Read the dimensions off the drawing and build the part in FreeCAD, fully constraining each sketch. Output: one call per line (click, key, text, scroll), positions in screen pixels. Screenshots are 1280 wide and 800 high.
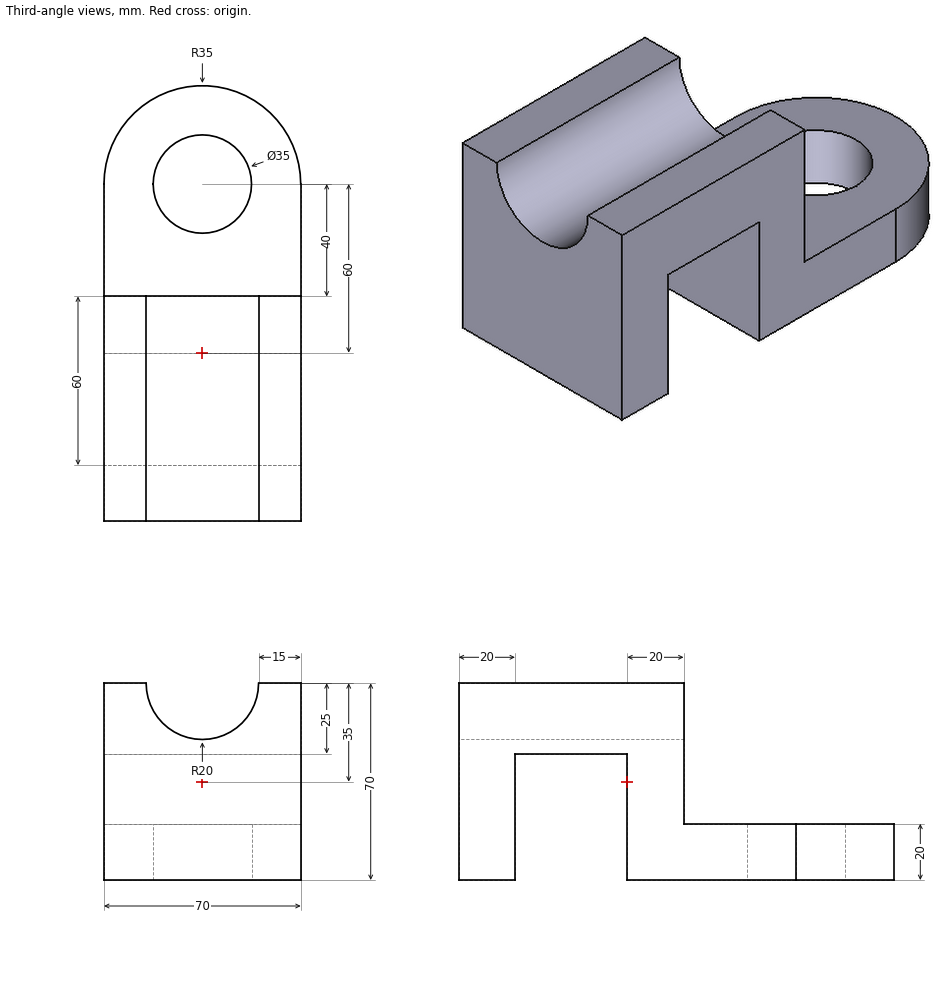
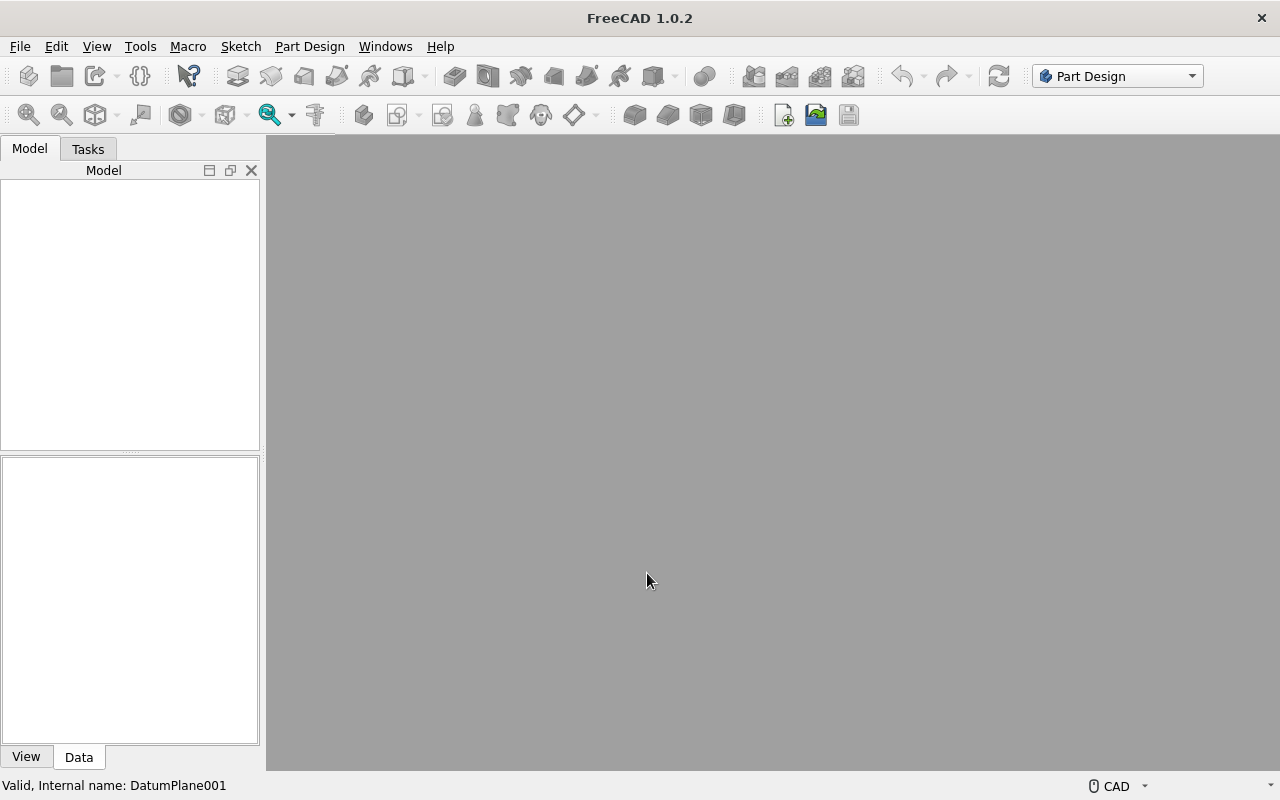
click(783, 116)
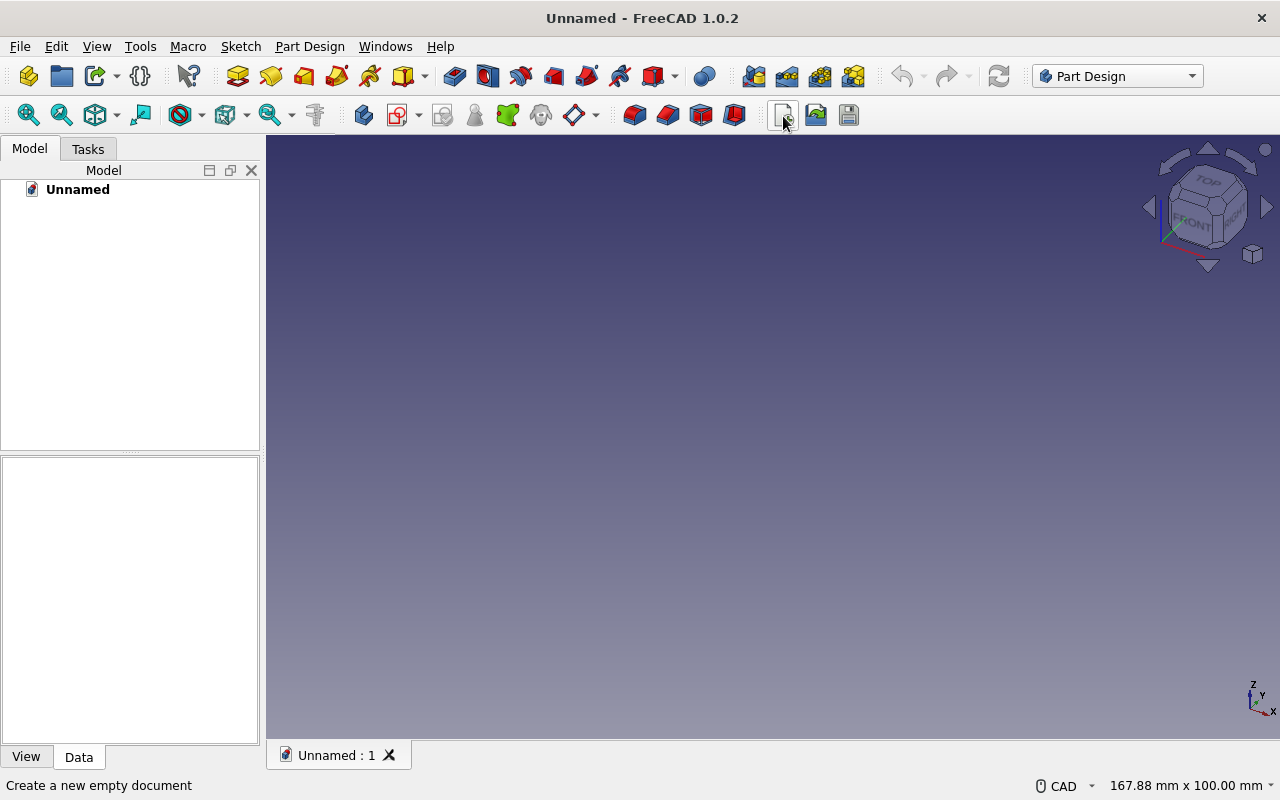
click(396, 116)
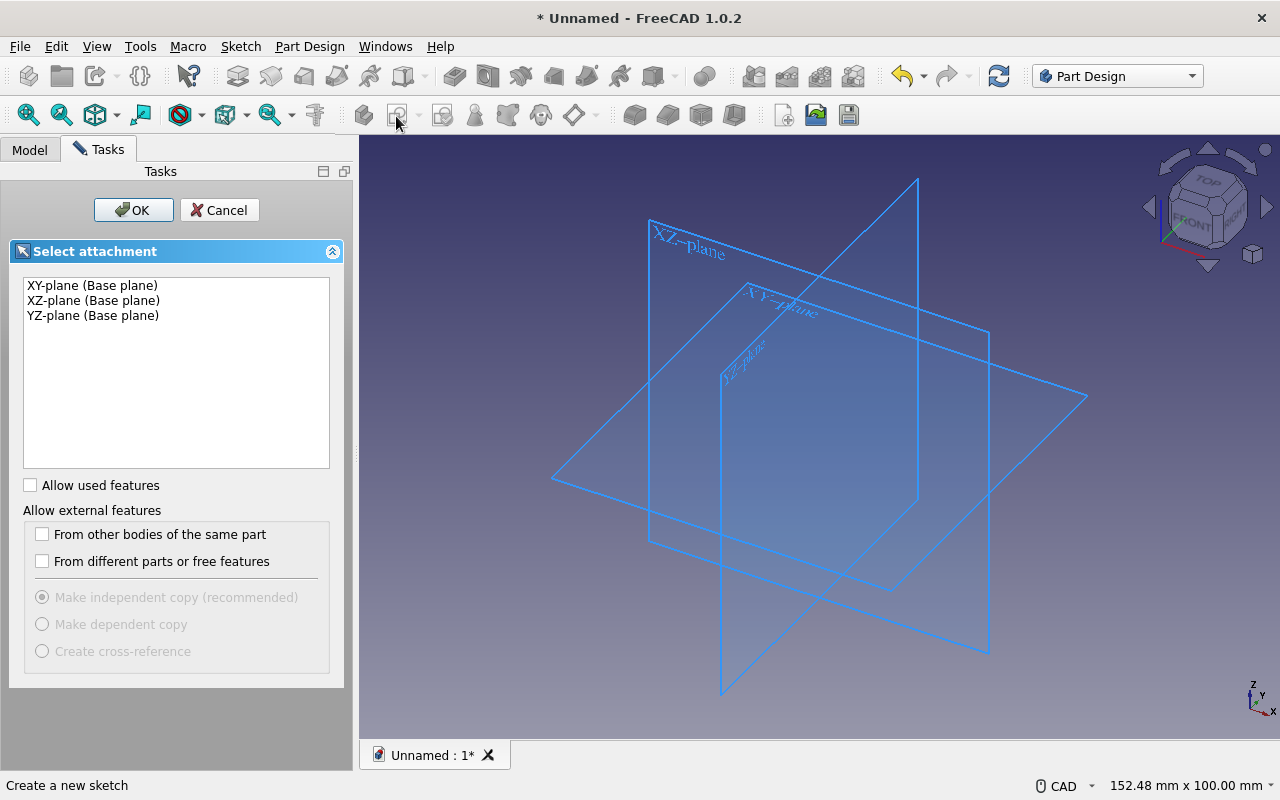
click(84, 300)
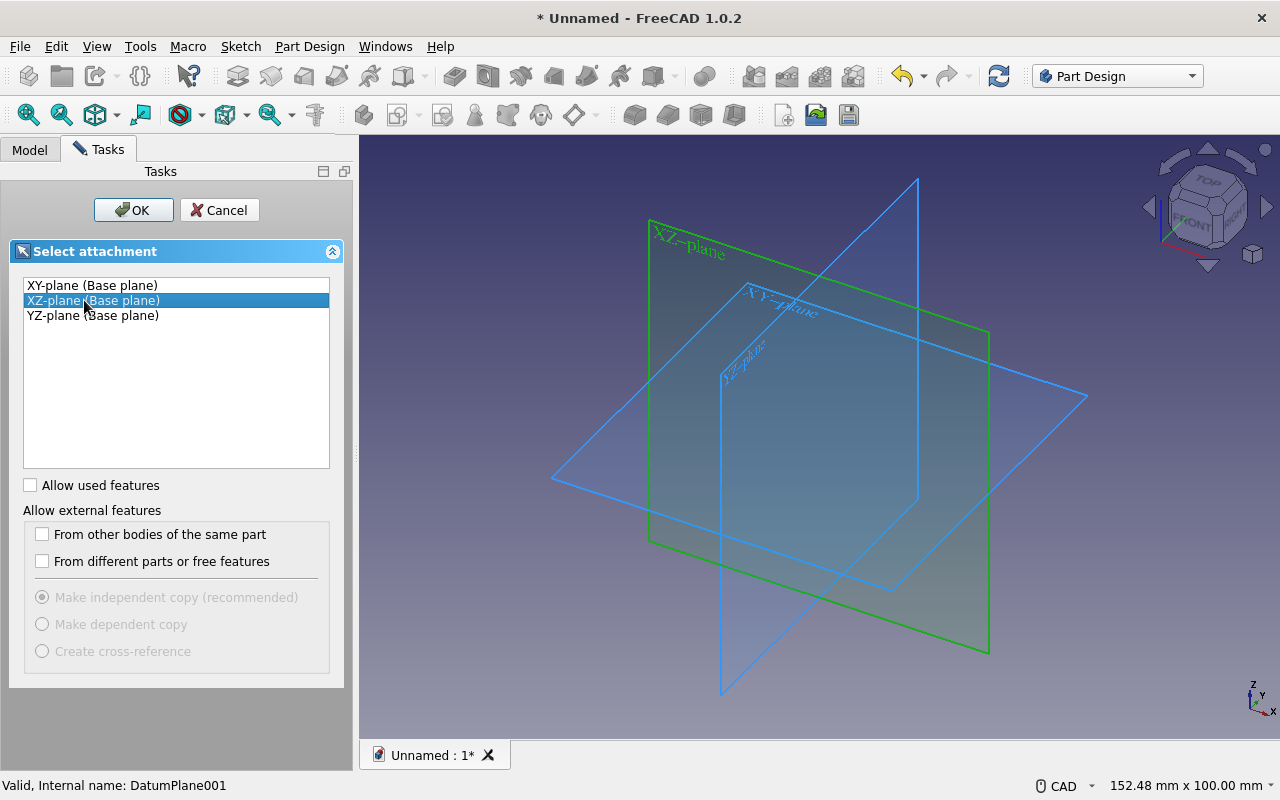
click(134, 210)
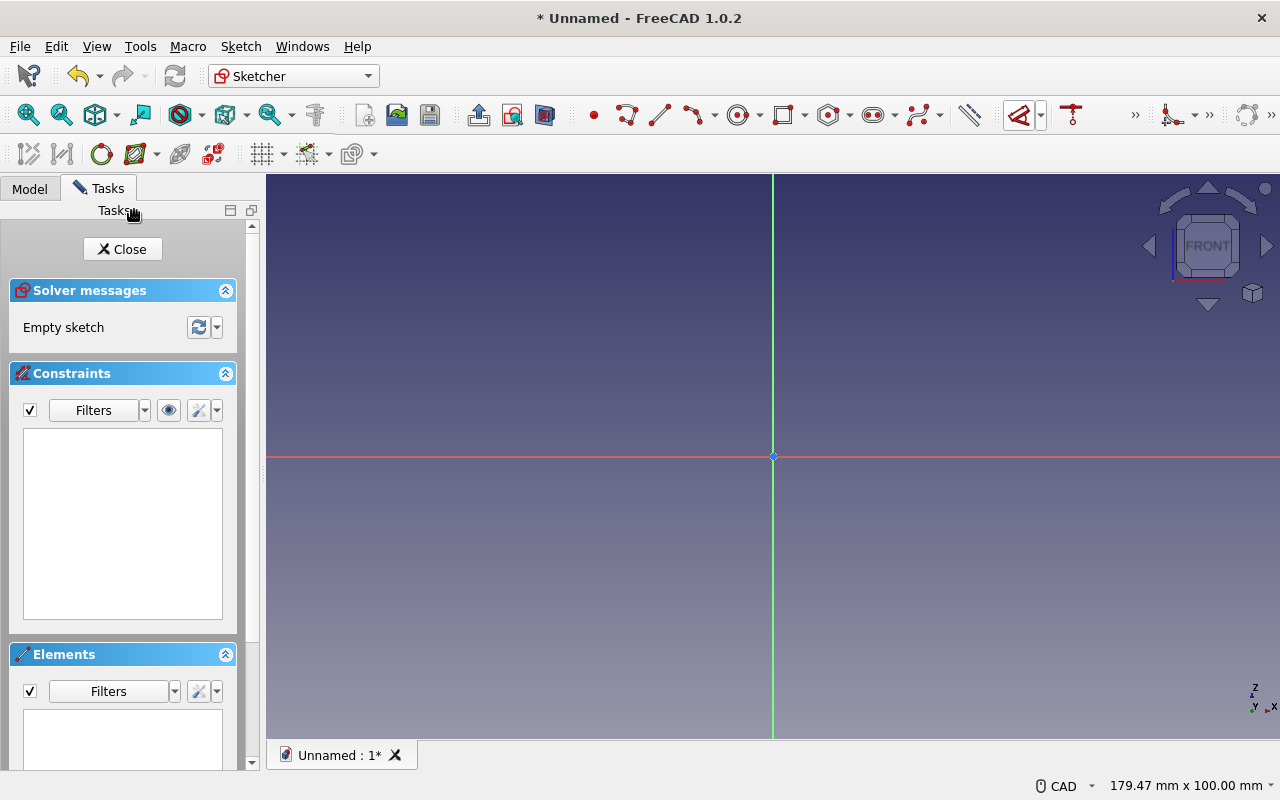
click(627, 116)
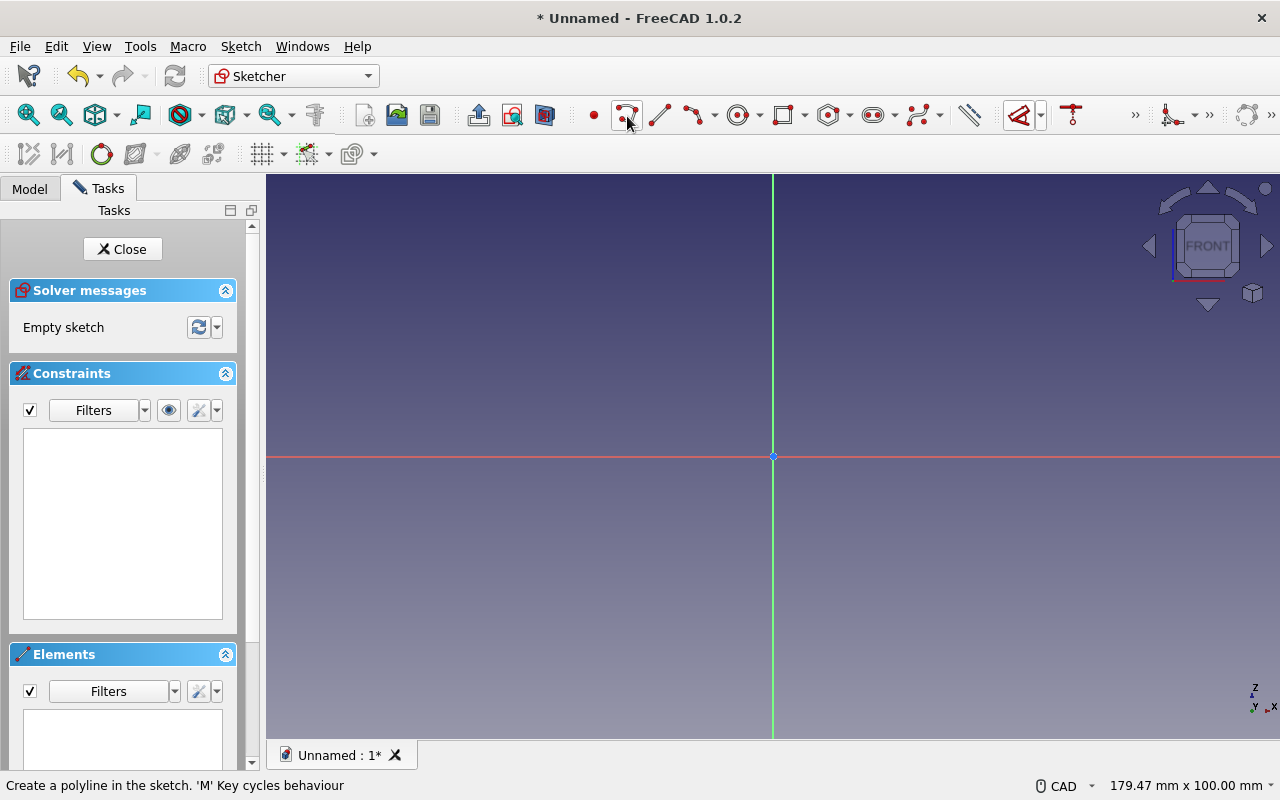
click(886, 259)
click(971, 259)
click(971, 654)
click(575, 654)
click(575, 259)
click(660, 259)
right_click(660, 259)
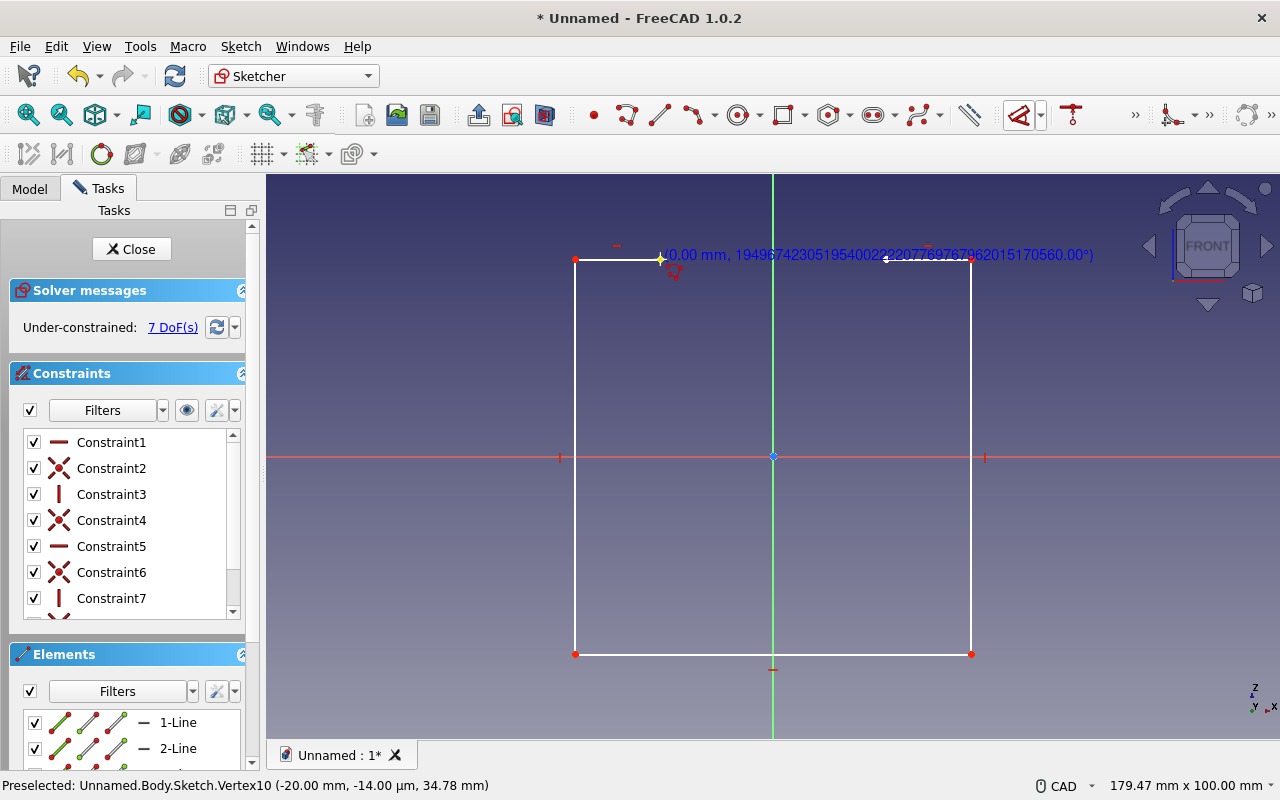
key(g)
key(3)
key(a)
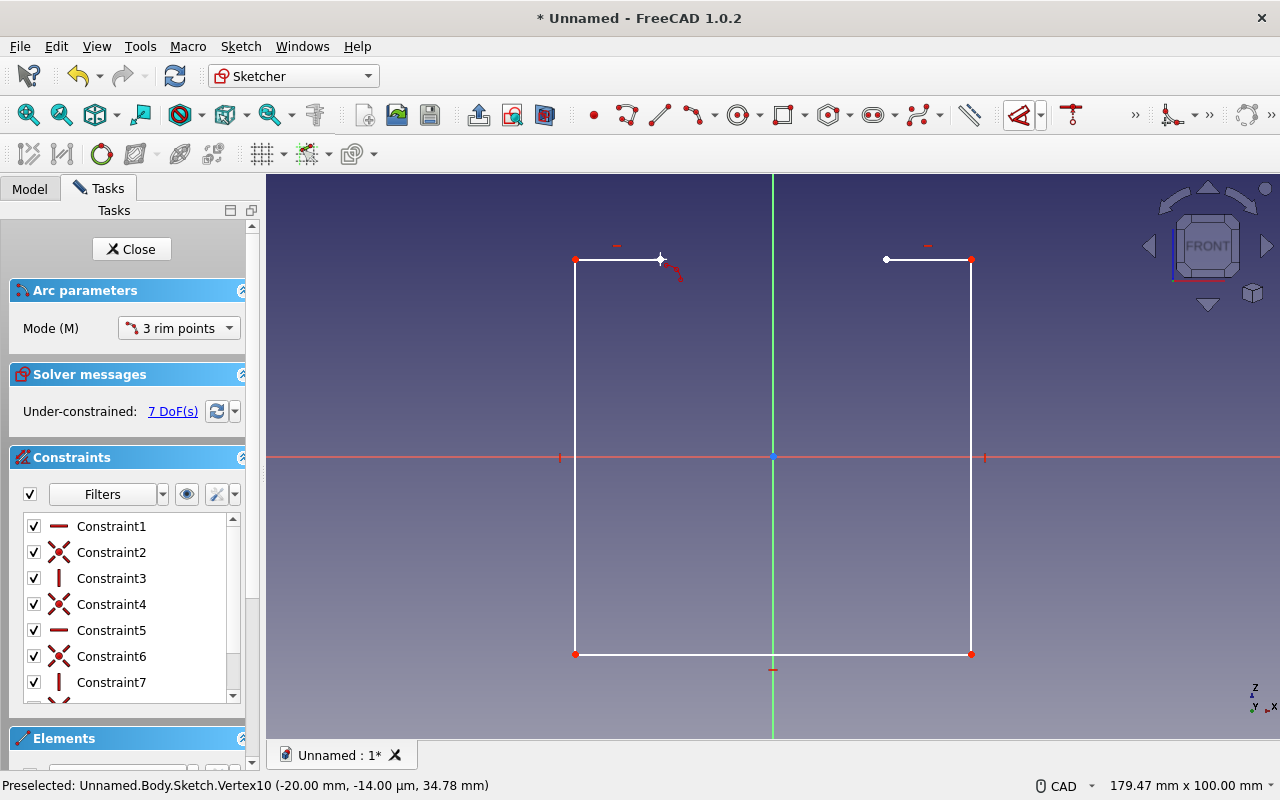
click(660, 260)
click(886, 260)
click(738, 366)
key(Escape)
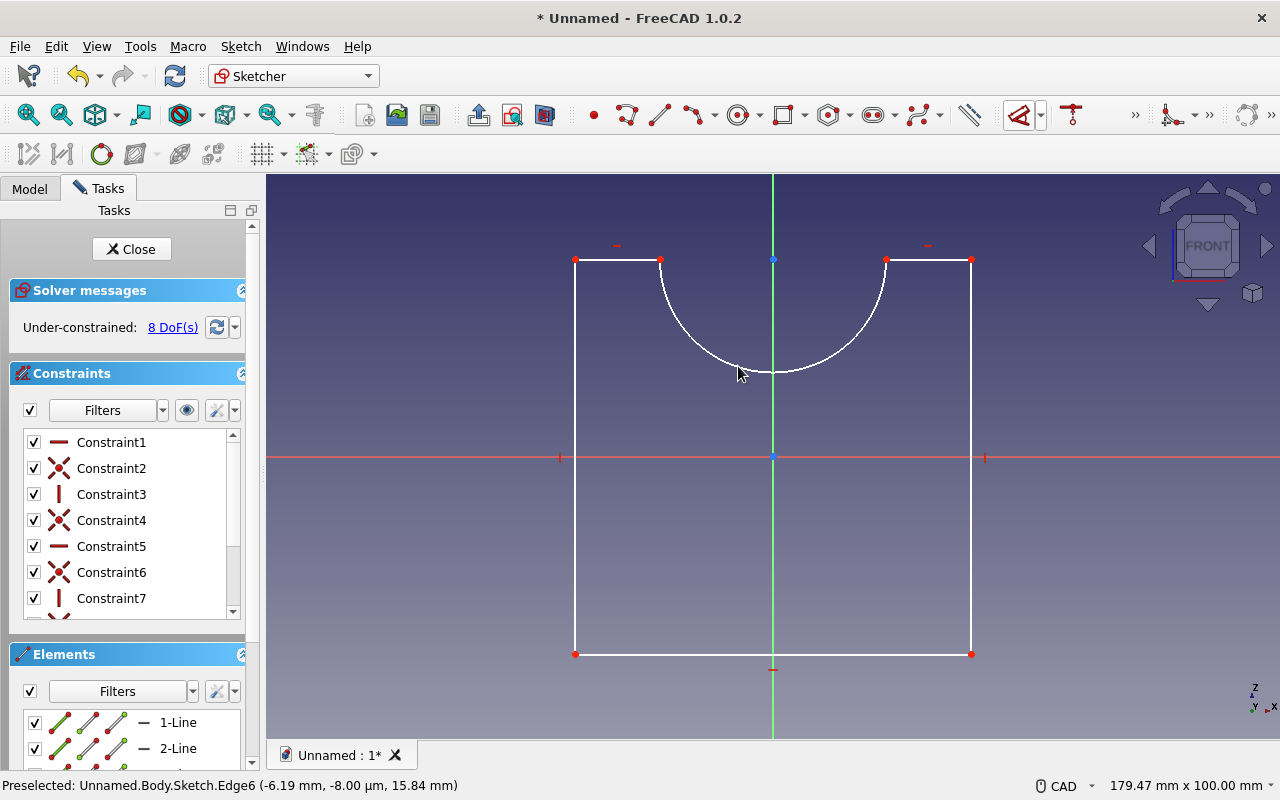
click(773, 260)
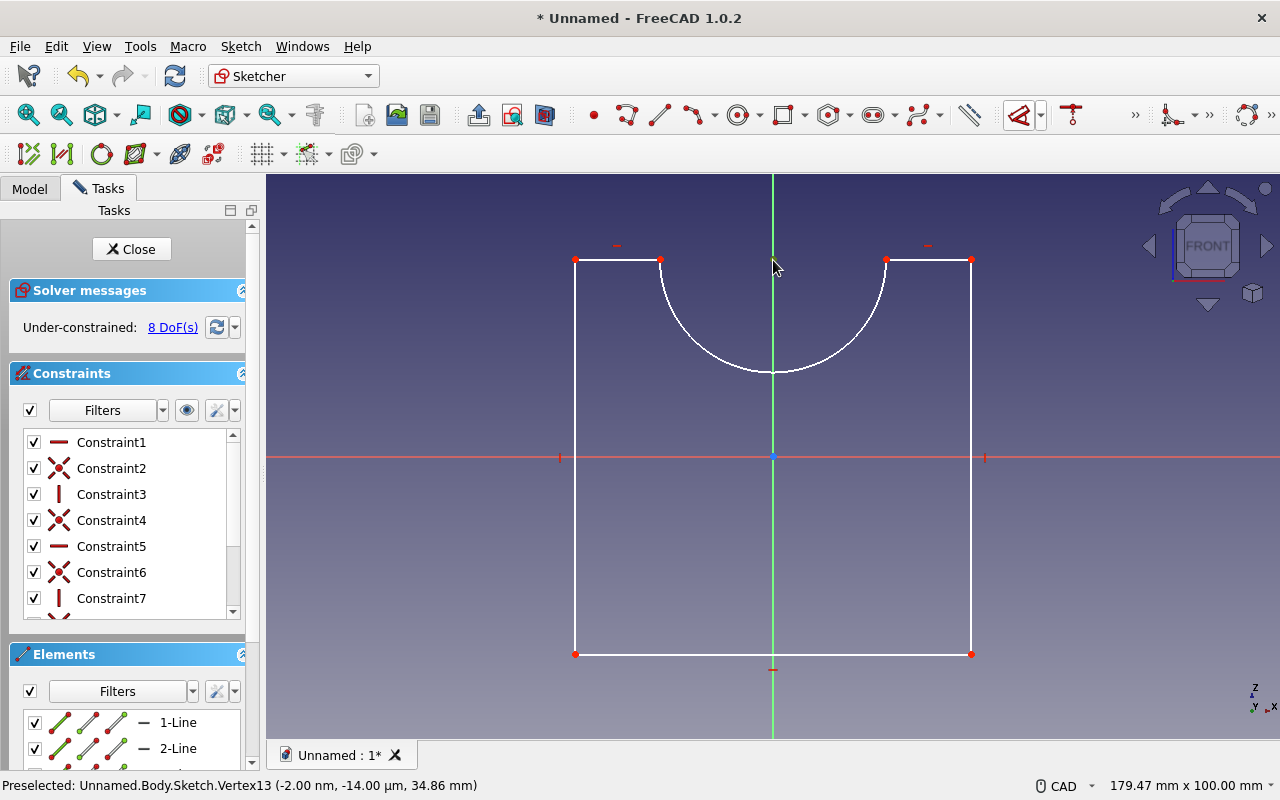
click(773, 602)